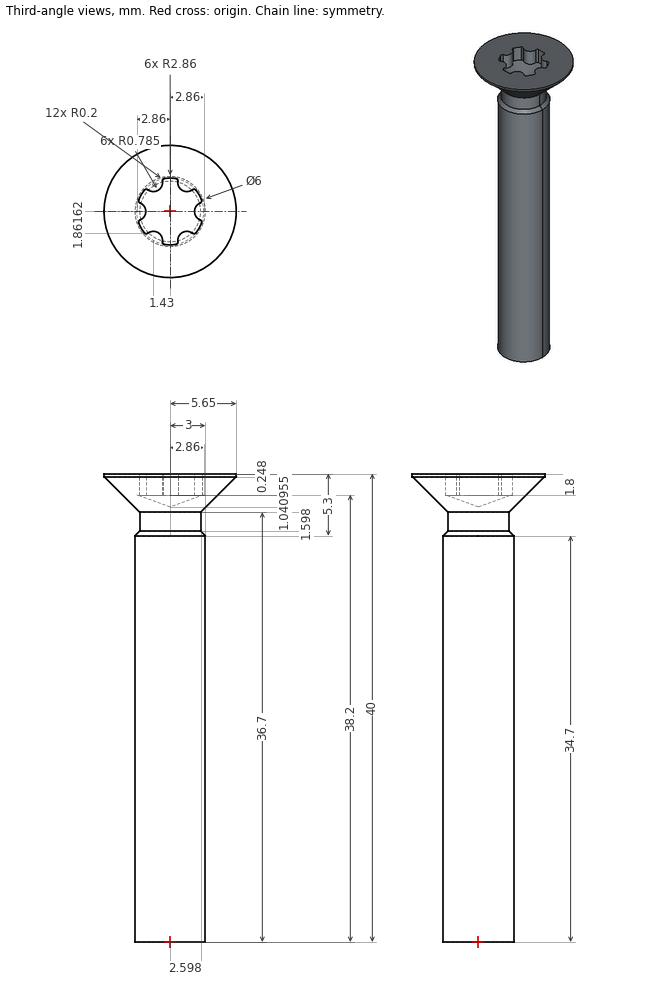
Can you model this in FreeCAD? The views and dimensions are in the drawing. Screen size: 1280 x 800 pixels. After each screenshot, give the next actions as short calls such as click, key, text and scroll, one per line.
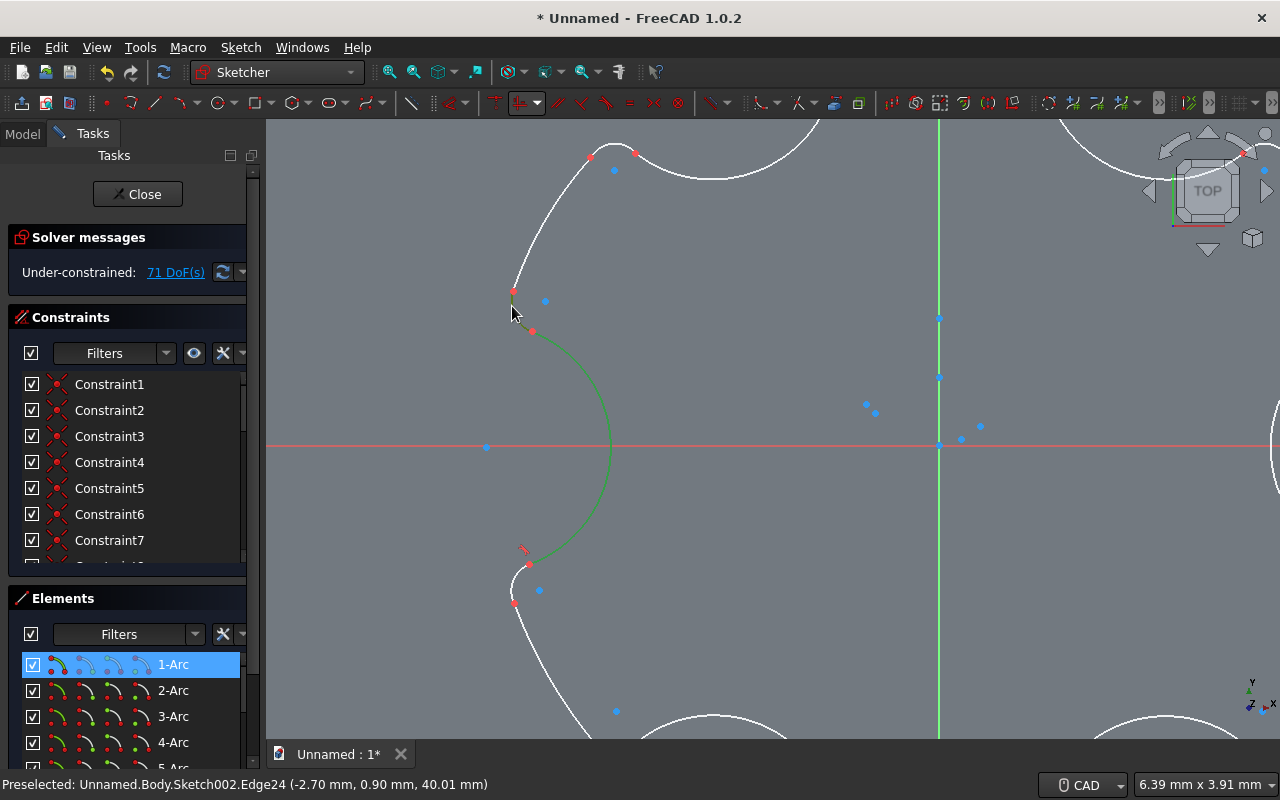
click(606, 104)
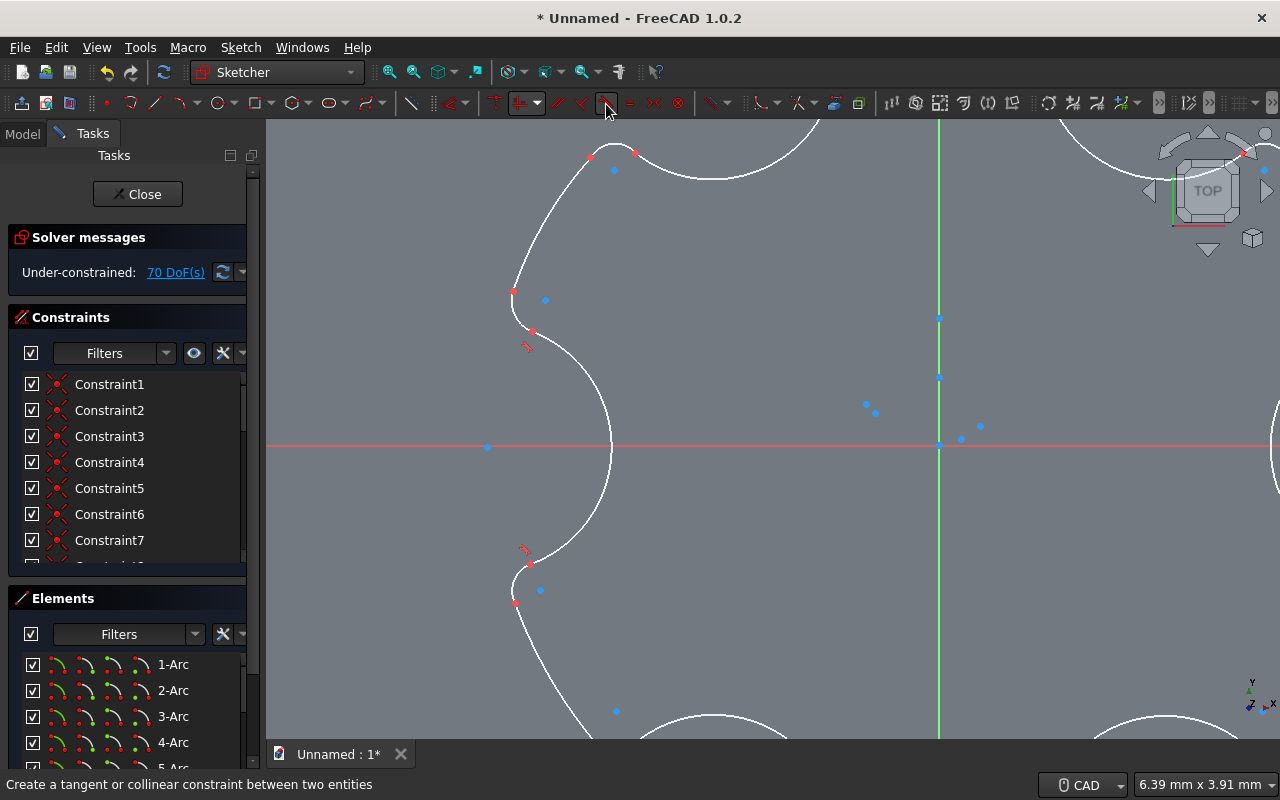
click(519, 572)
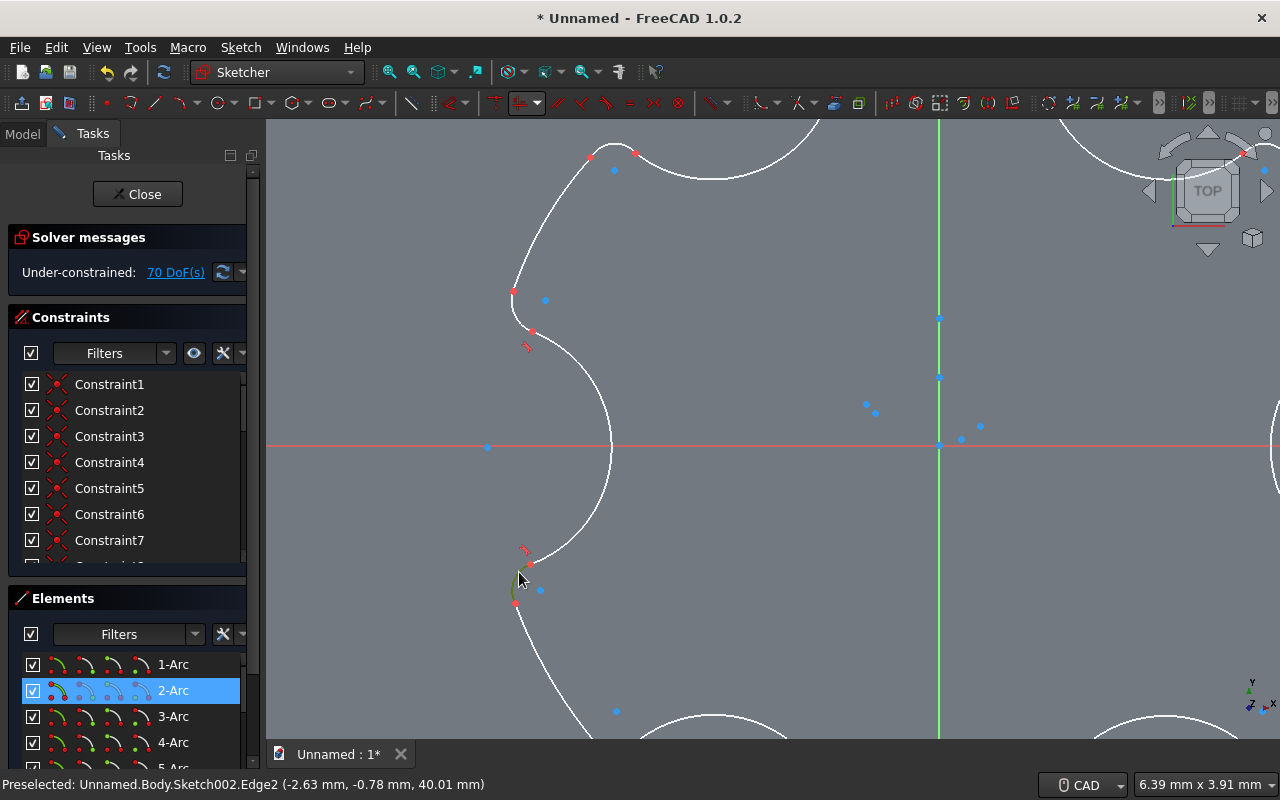
click(533, 647)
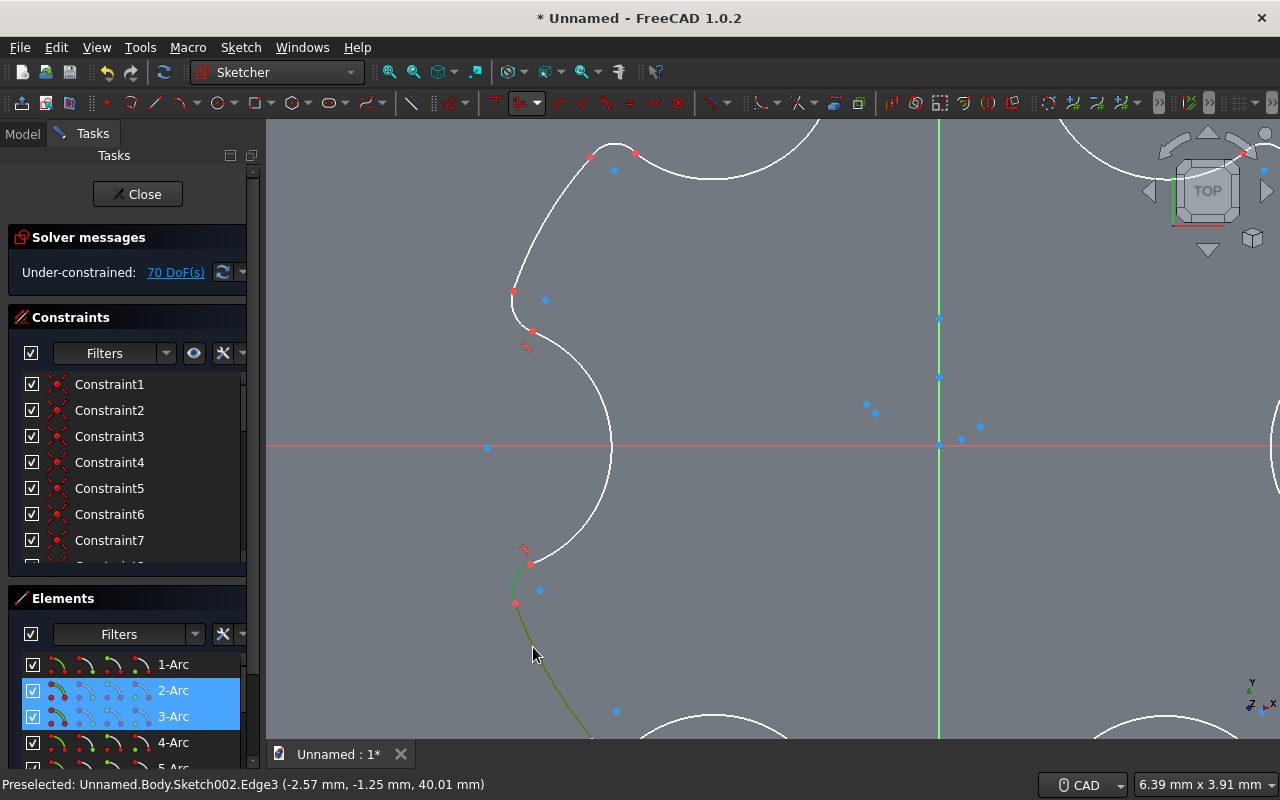
click(606, 104)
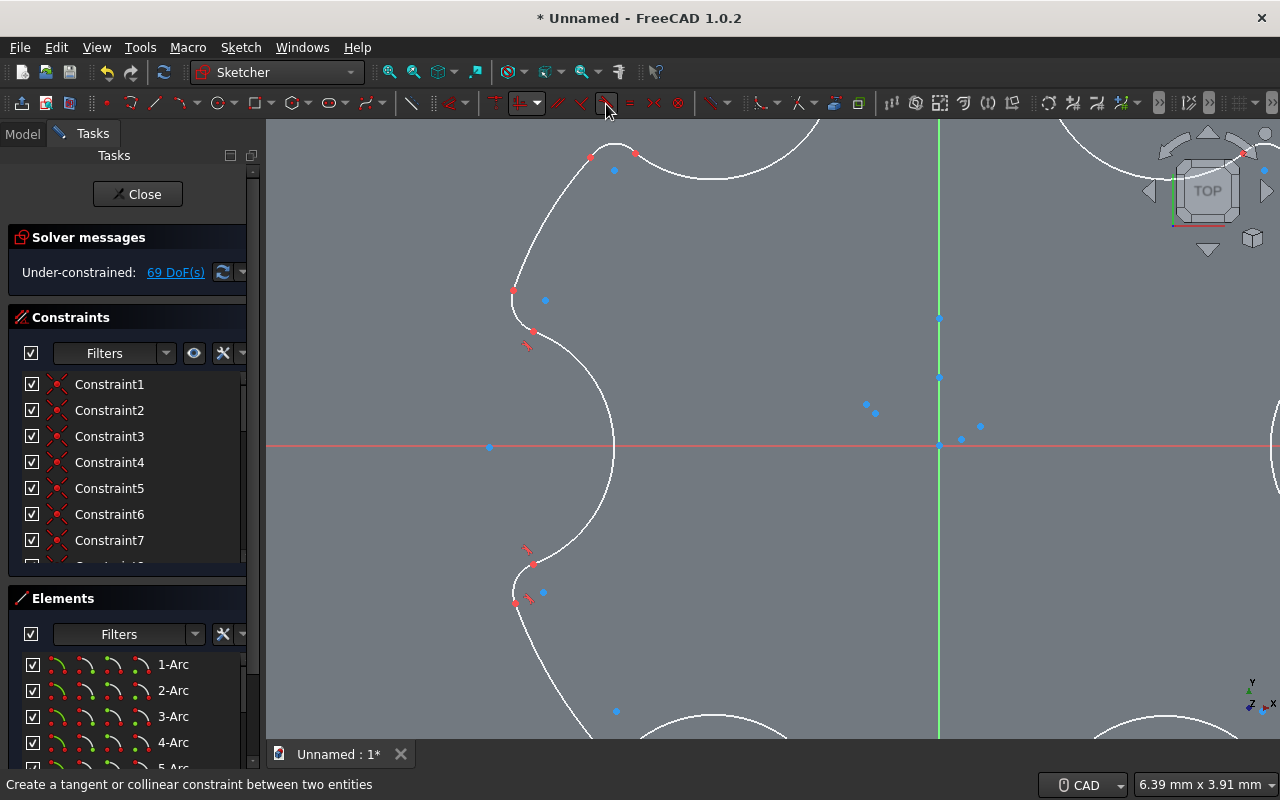
click(533, 646)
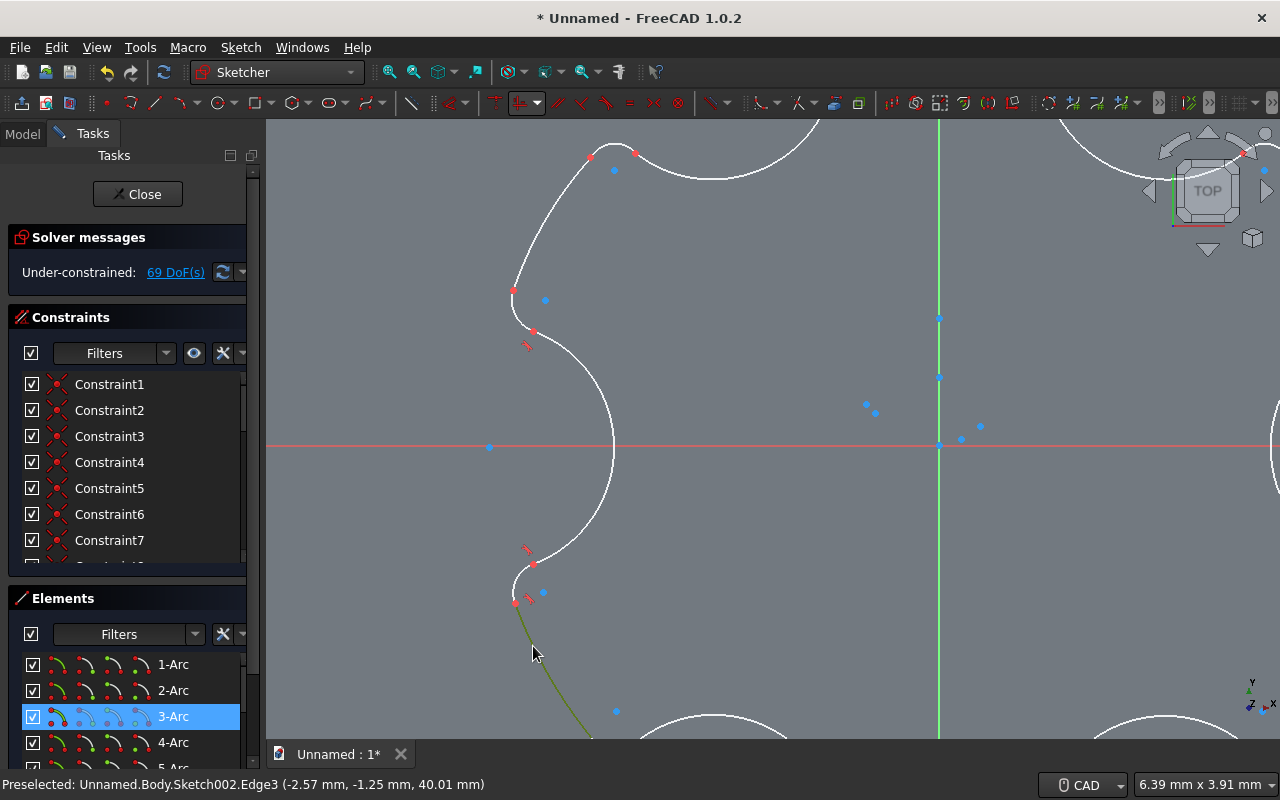
scroll(513, 416, down, 4)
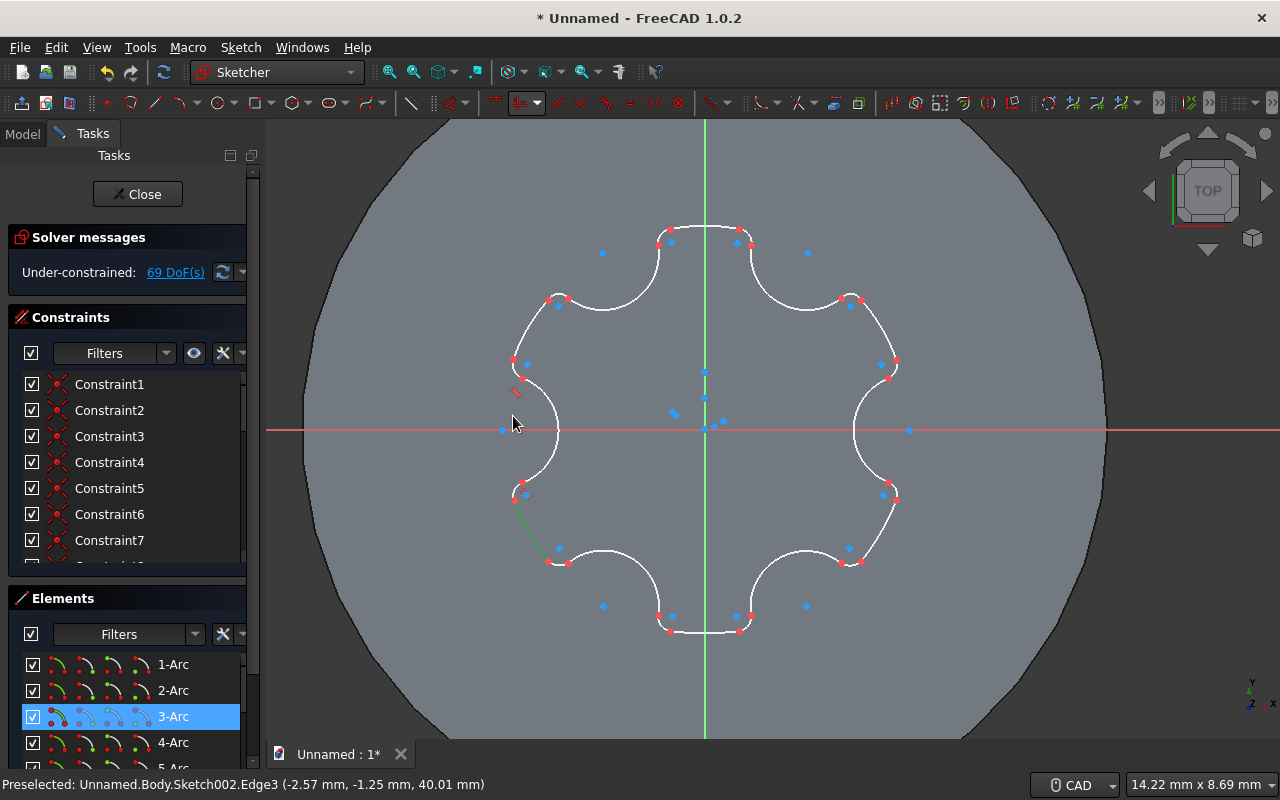
scroll(554, 564, up, 4)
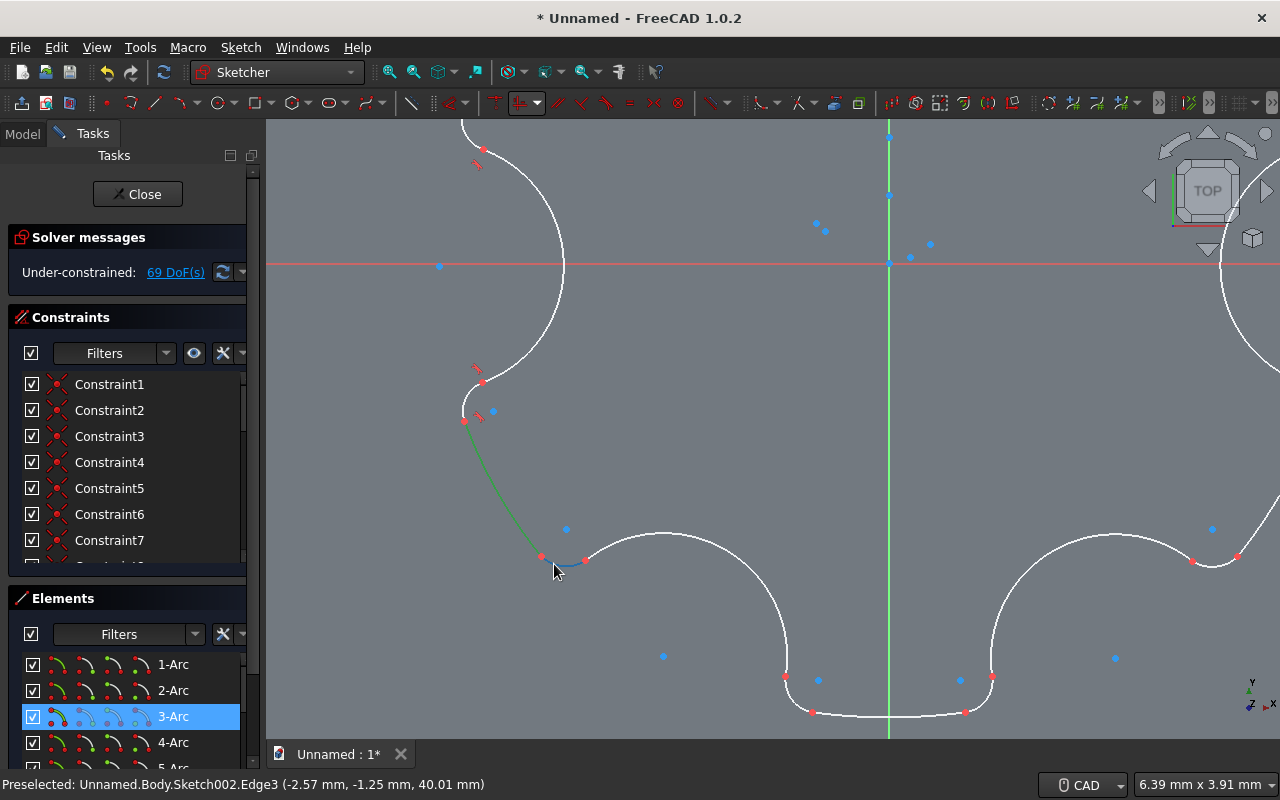
click(553, 564)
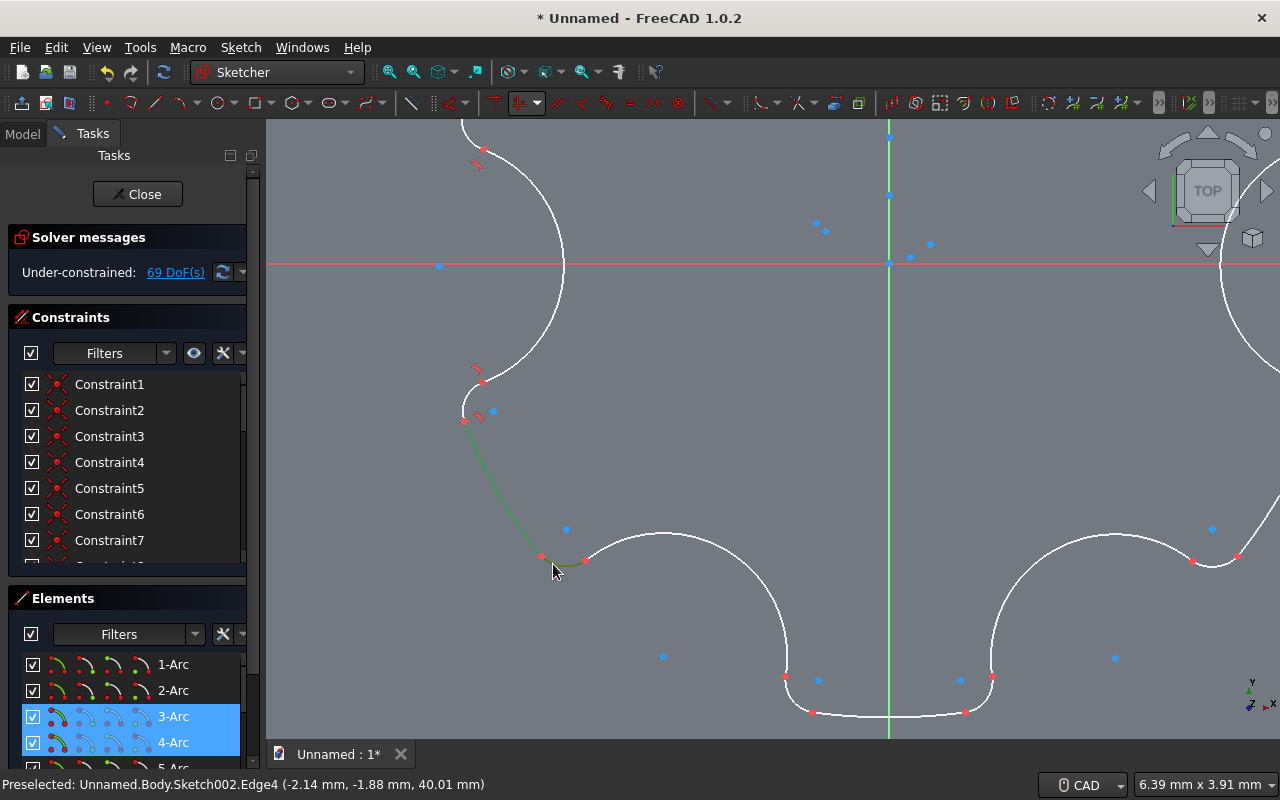
click(606, 104)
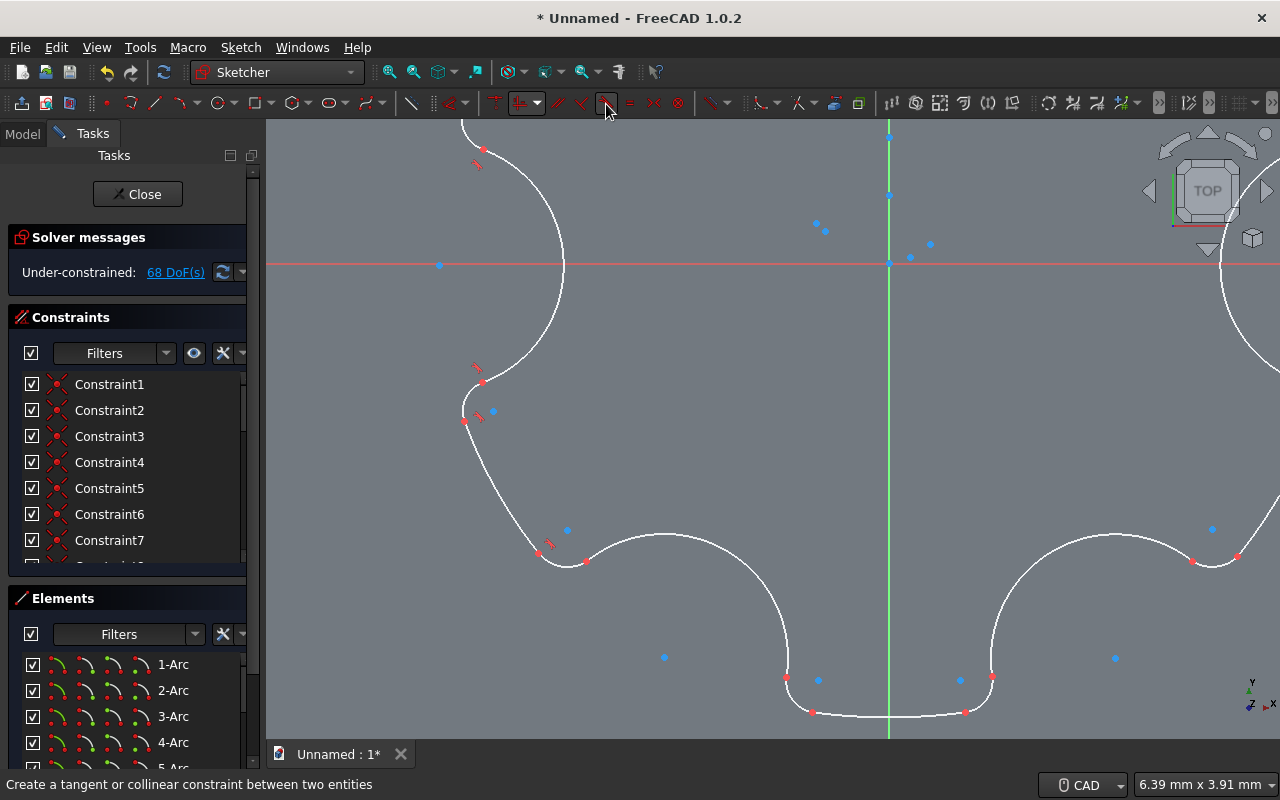
click(551, 563)